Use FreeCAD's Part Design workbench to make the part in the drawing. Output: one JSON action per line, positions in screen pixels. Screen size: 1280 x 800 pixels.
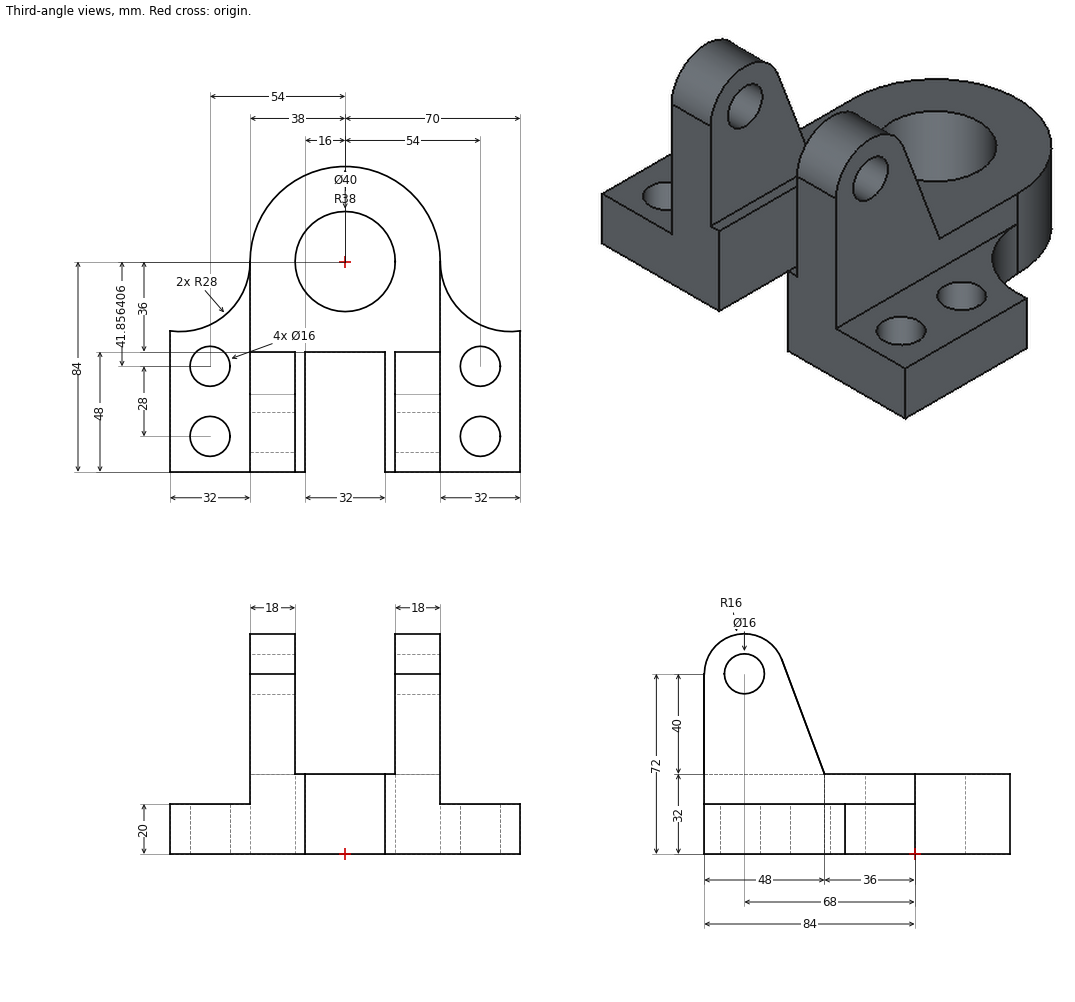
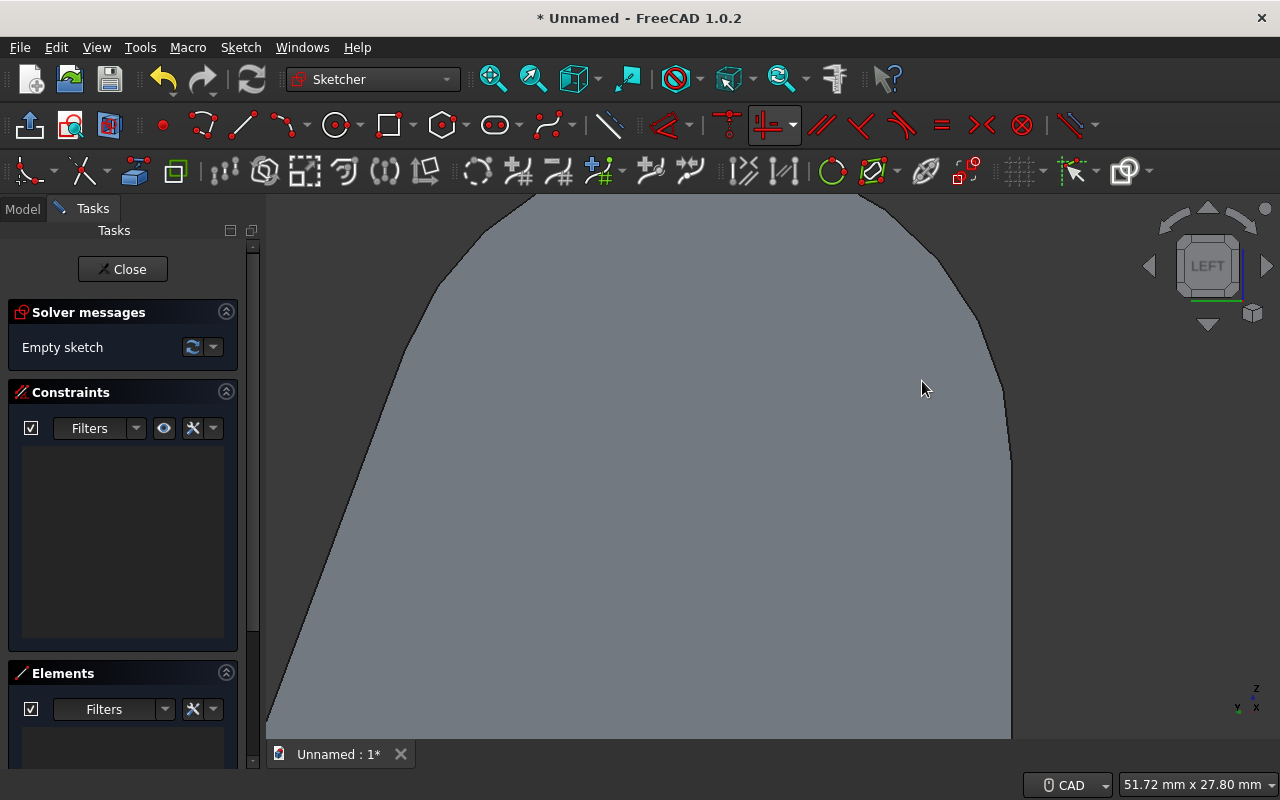
{"action": "left_click", "coordinate": [336, 126]}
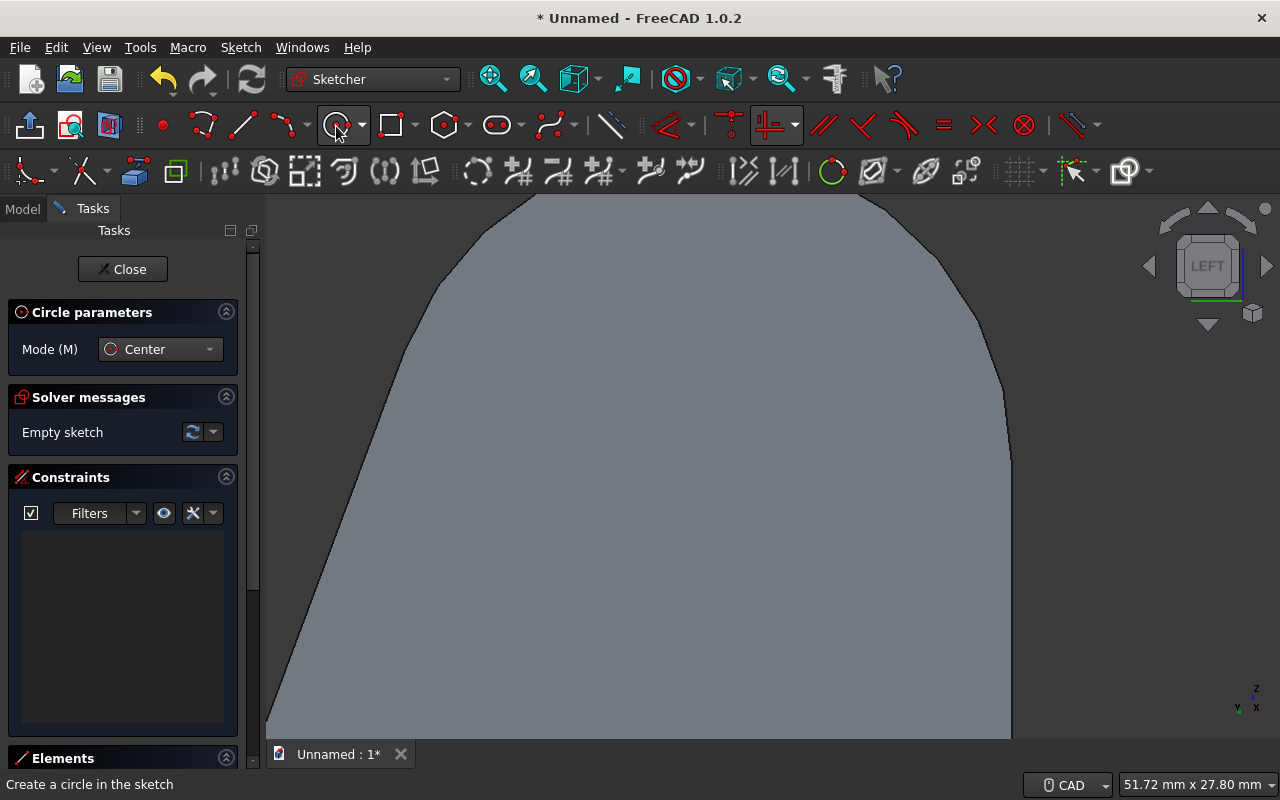
{"action": "left_click", "coordinate": [698, 461]}
{"action": "left_click", "coordinate": [809, 351]}
{"action": "key", "text": "Escape"}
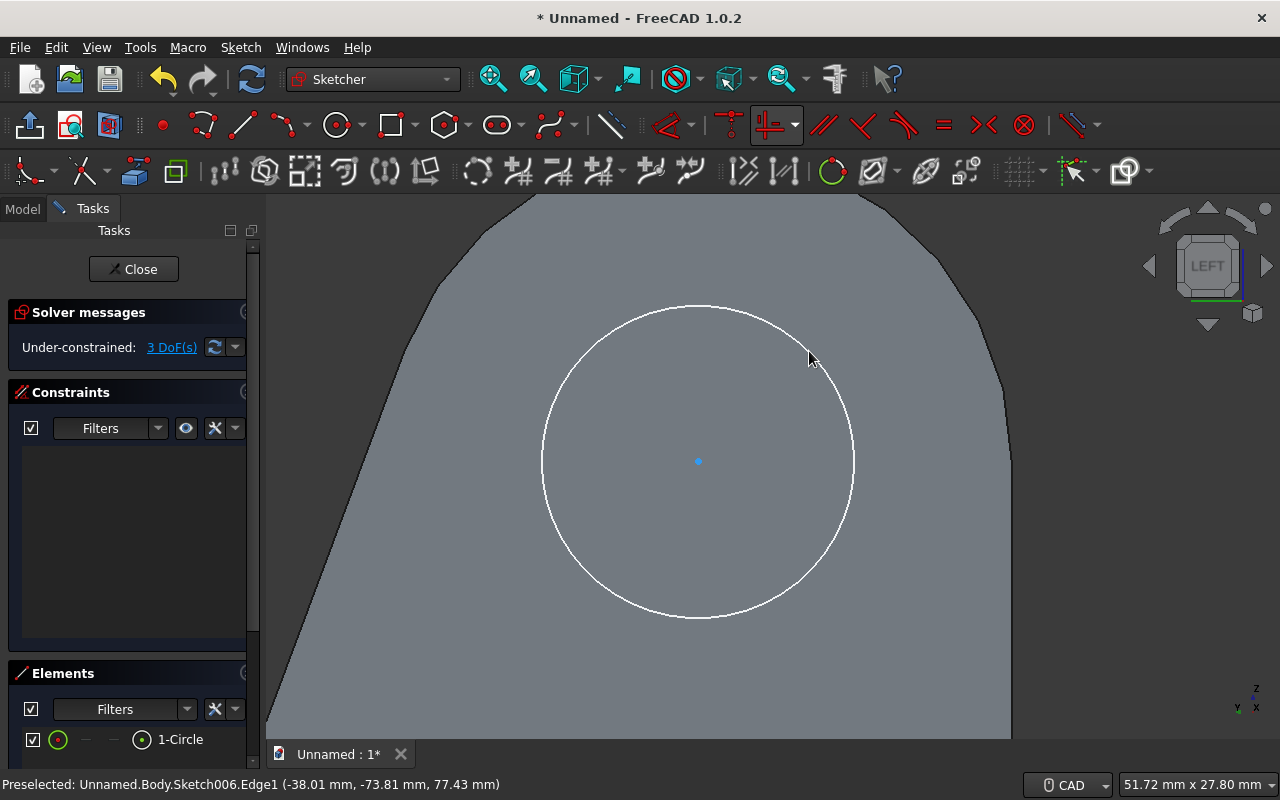
{"action": "left_click", "coordinate": [666, 126]}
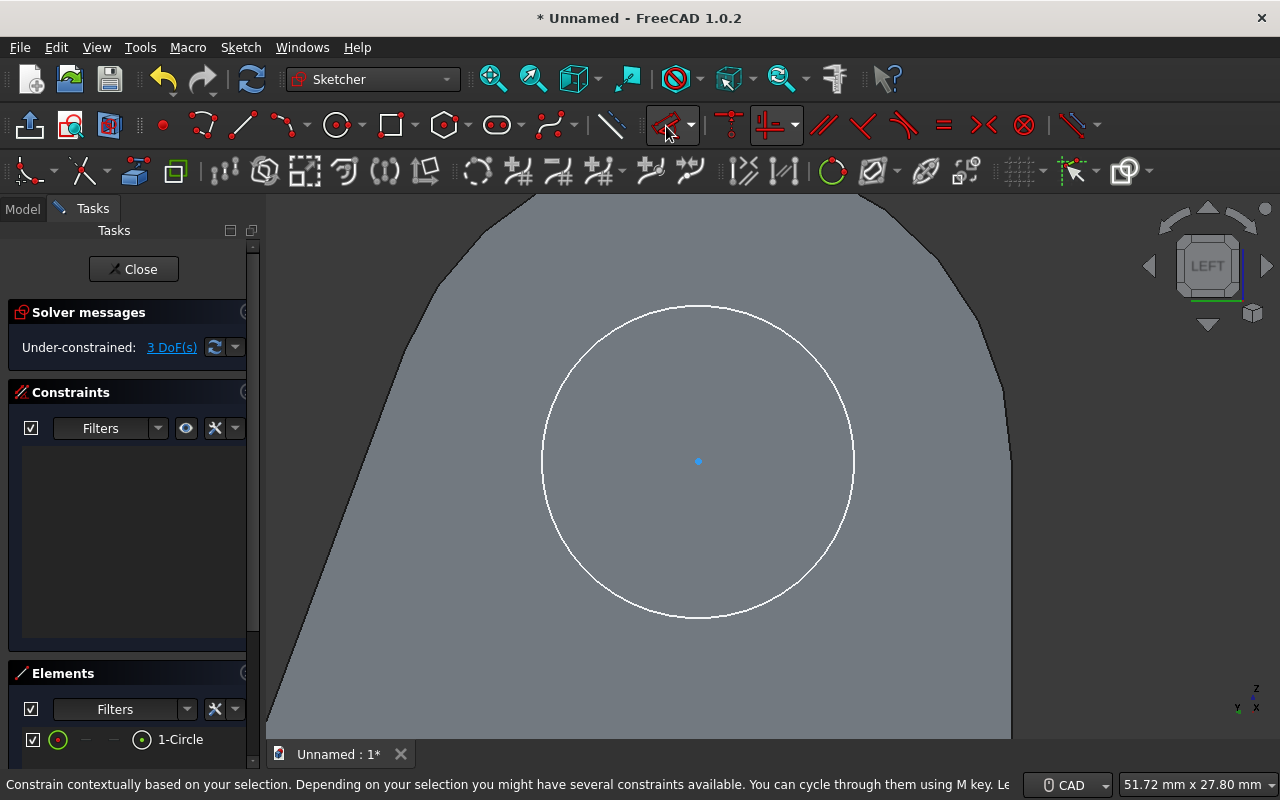
{"action": "left_click", "coordinate": [808, 351]}
{"action": "left_click", "coordinate": [831, 328]}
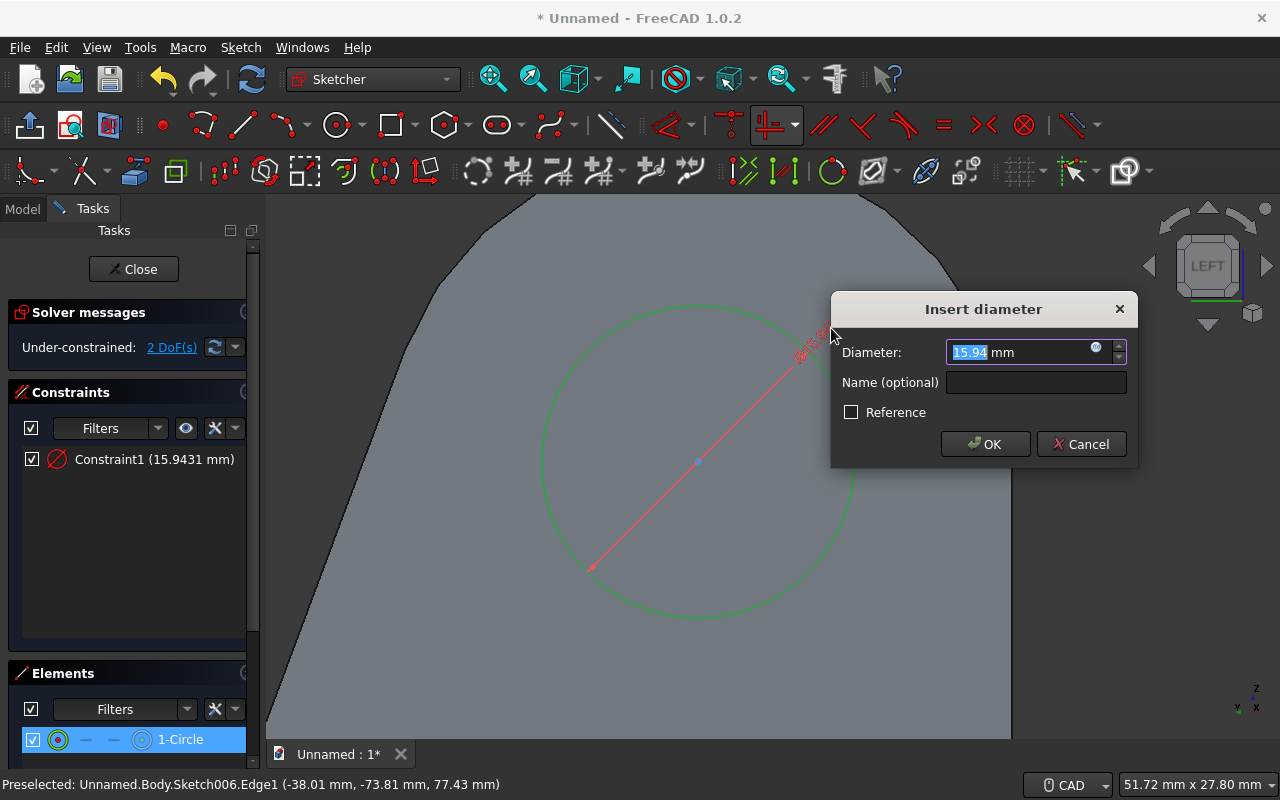
{"action": "type", "text": "16"}
{"action": "key", "text": "Return"}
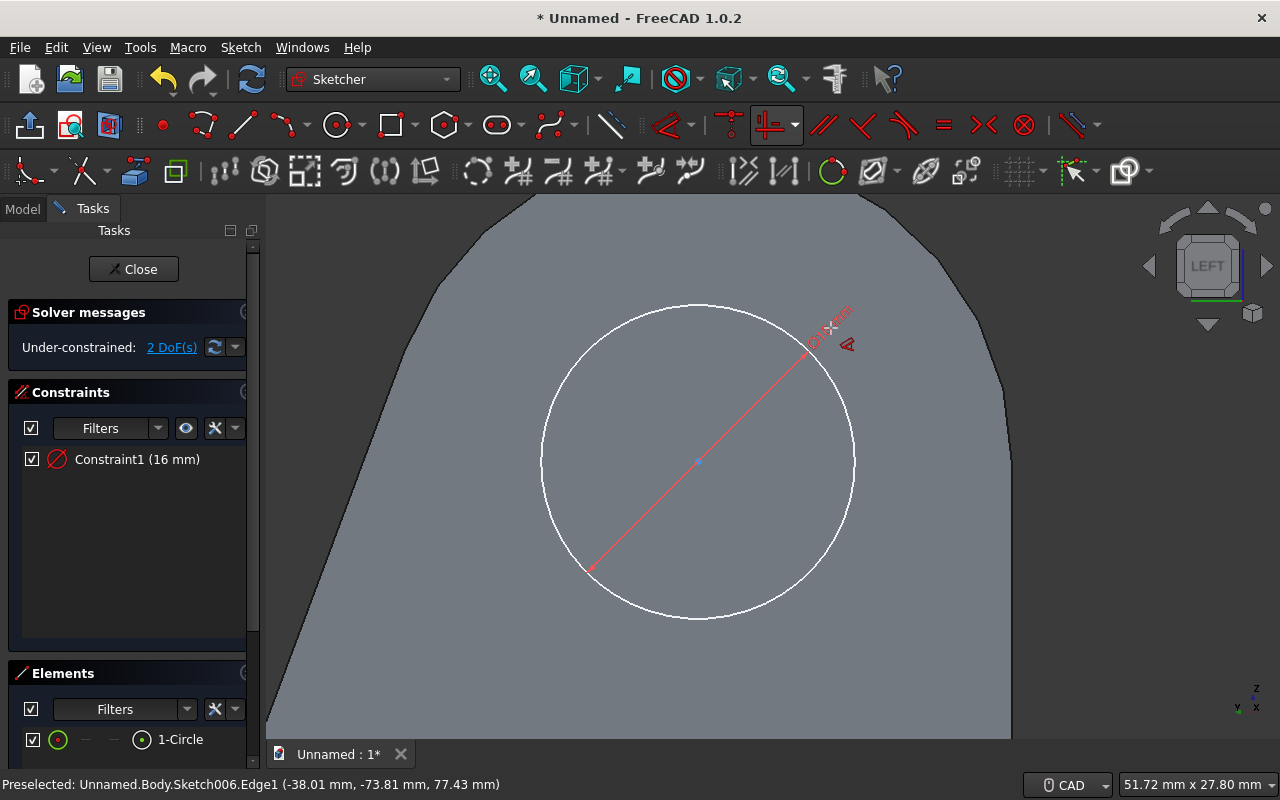
{"action": "left_click", "coordinate": [698, 462]}
{"action": "left_click", "coordinate": [496, 428]}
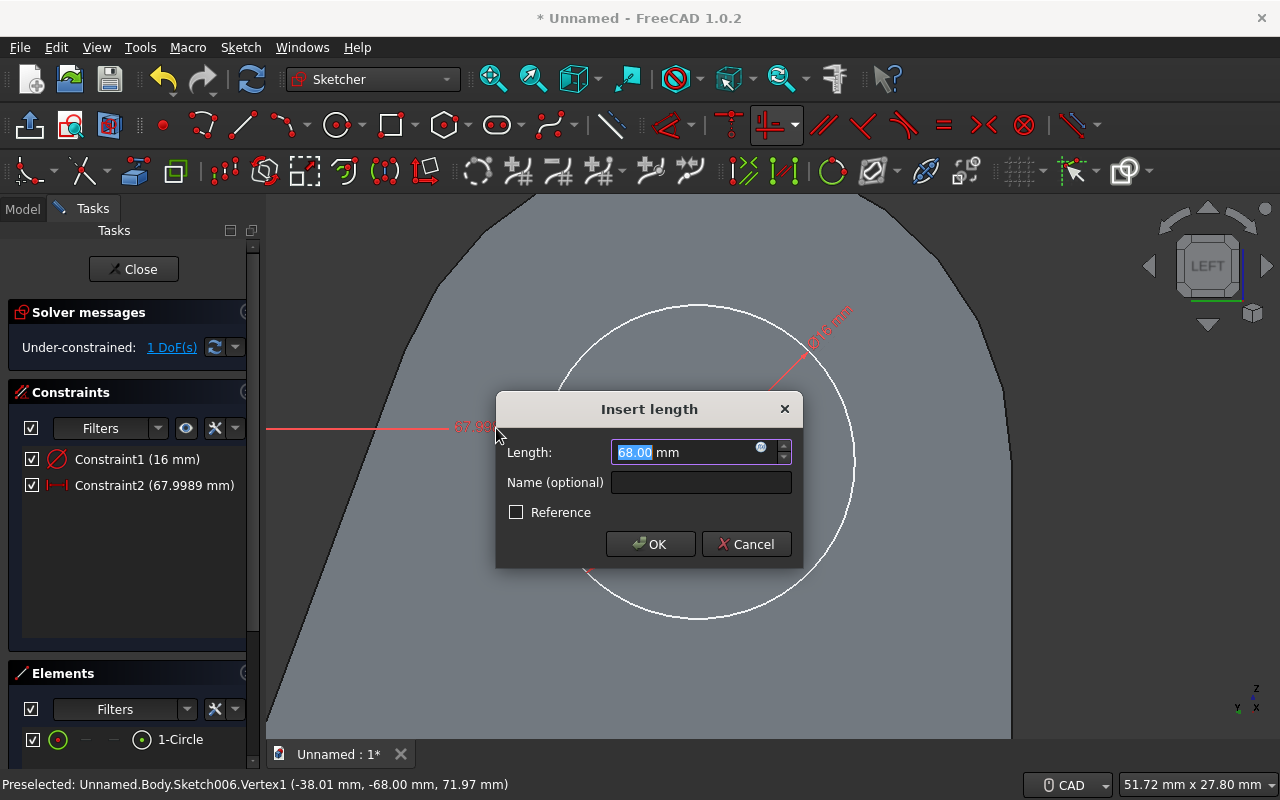
{"action": "type", "text": "68"}
{"action": "key", "text": "Return"}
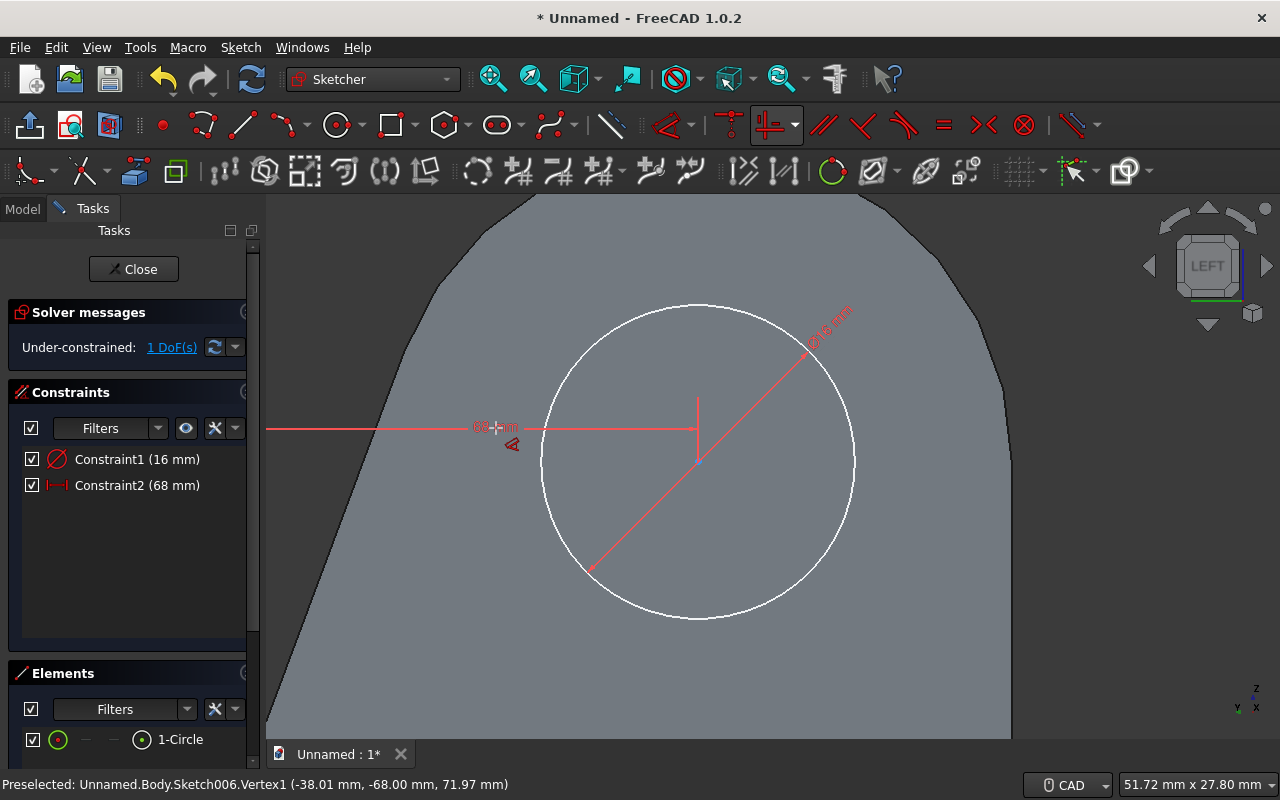
{"action": "left_click", "coordinate": [698, 462]}
{"action": "left_click", "coordinate": [732, 587]}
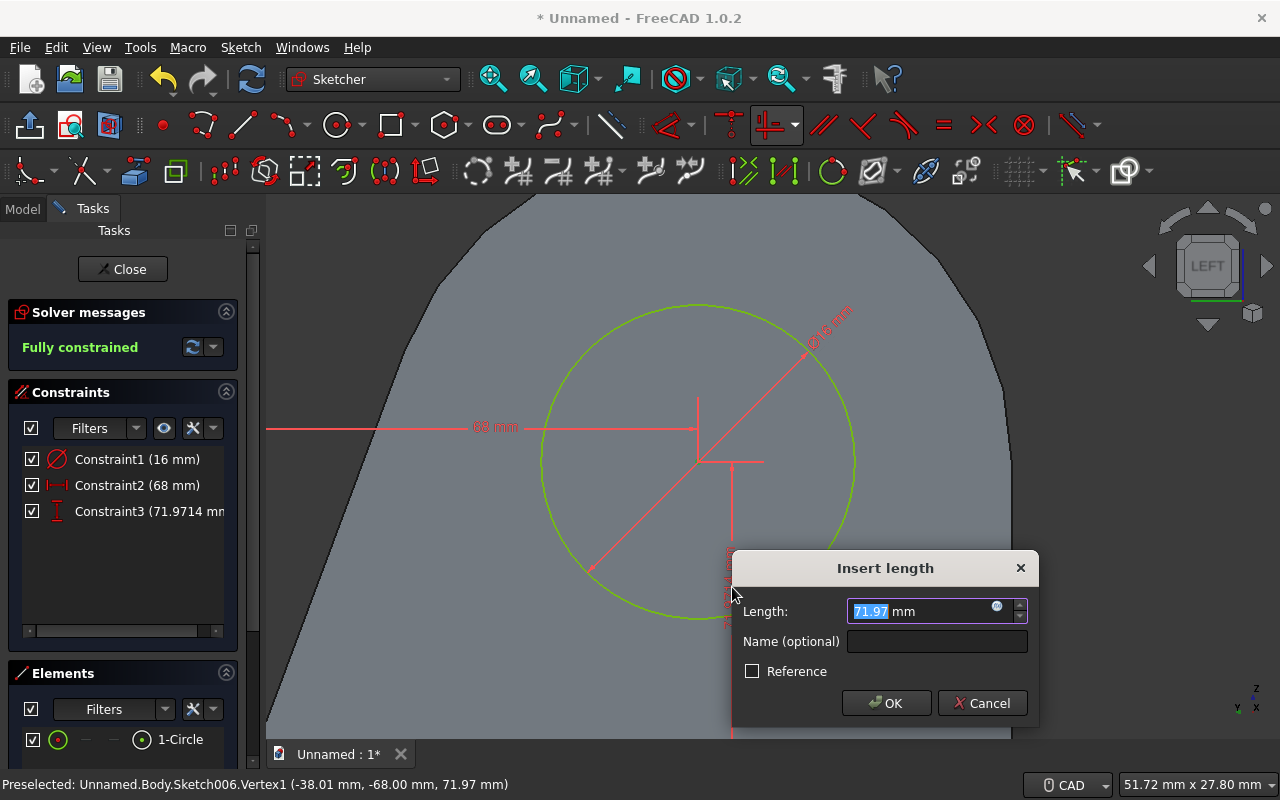
{"action": "type", "text": "72"}
{"action": "key", "text": "Return"}
{"action": "key", "text": "Escape"}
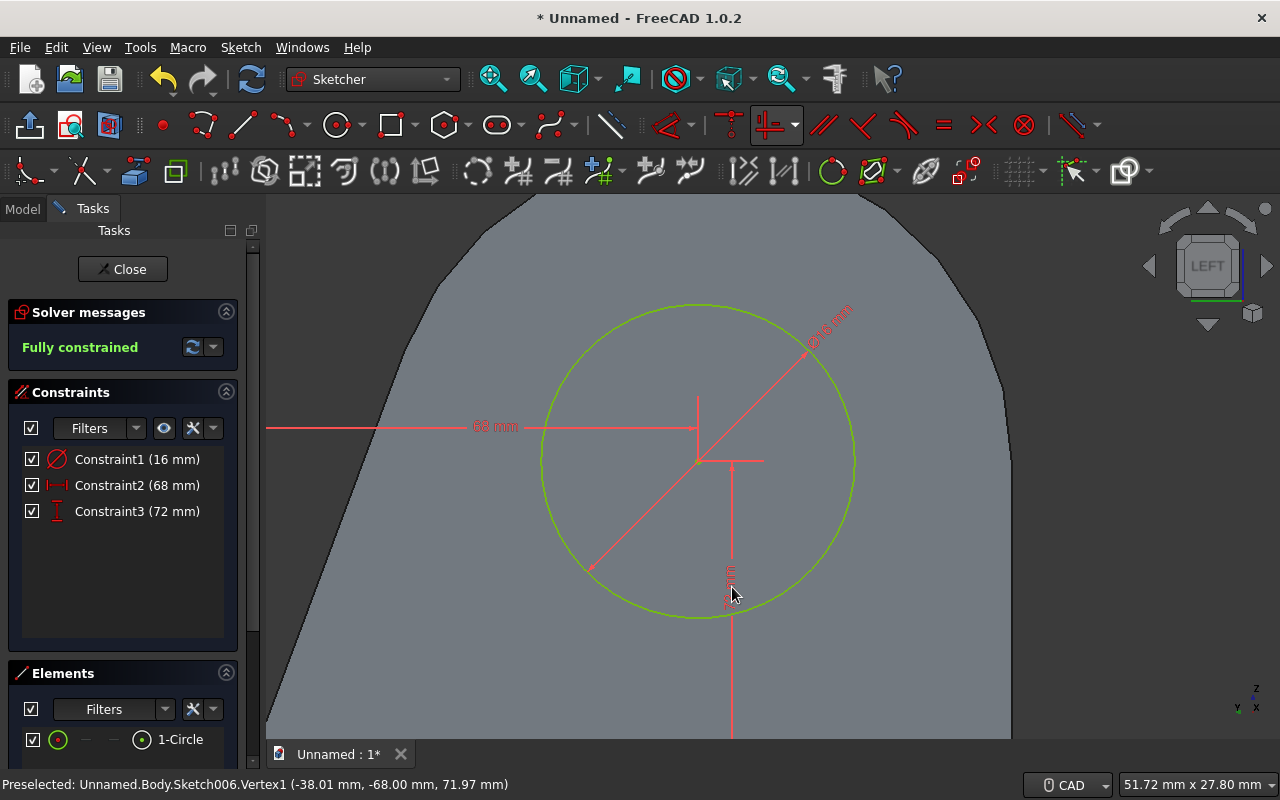
{"action": "left_click", "coordinate": [123, 269]}